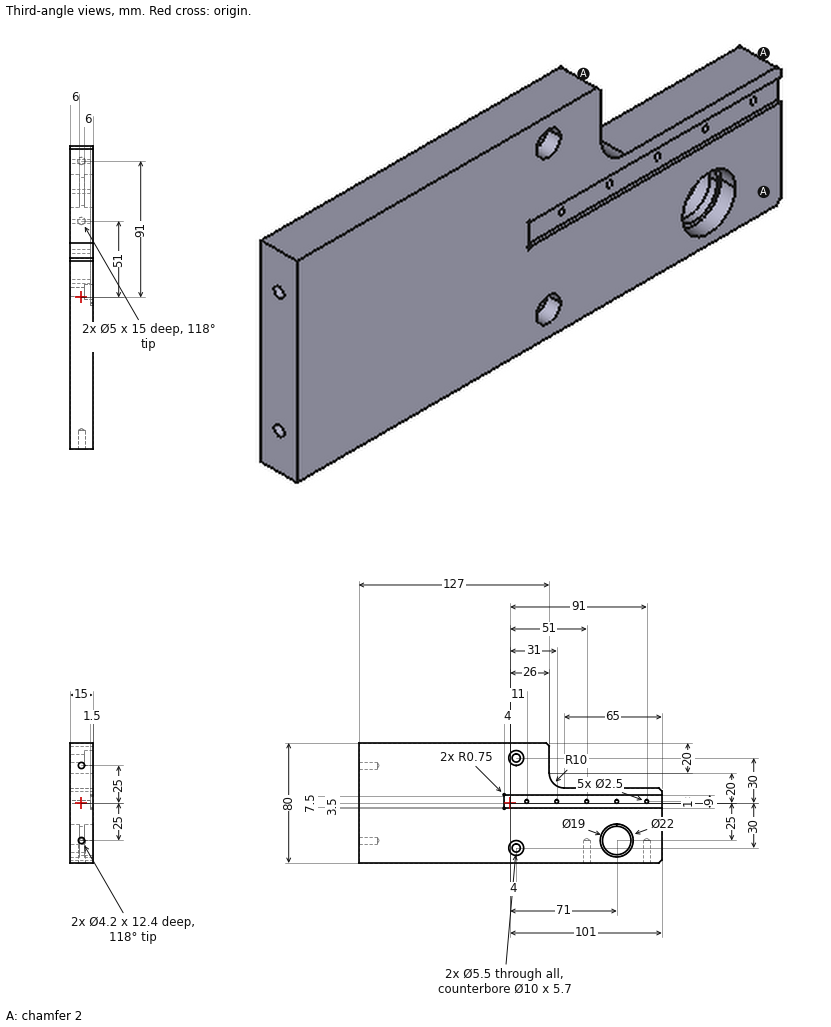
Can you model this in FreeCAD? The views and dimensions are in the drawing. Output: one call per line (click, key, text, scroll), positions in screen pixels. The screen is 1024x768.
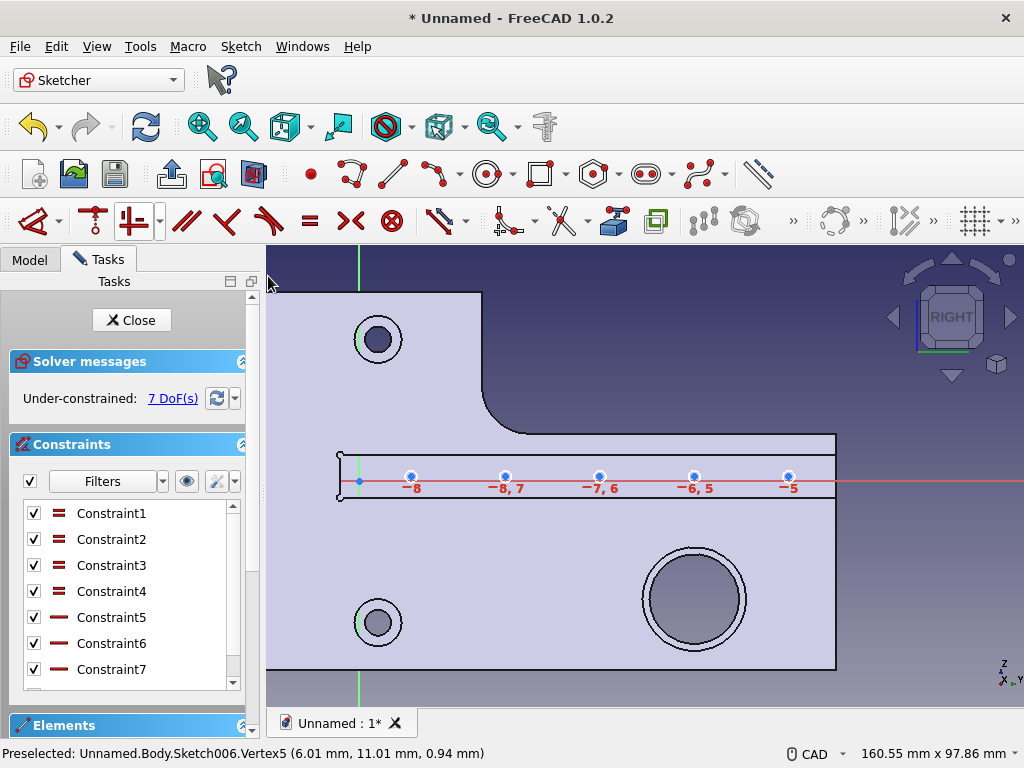
key(d)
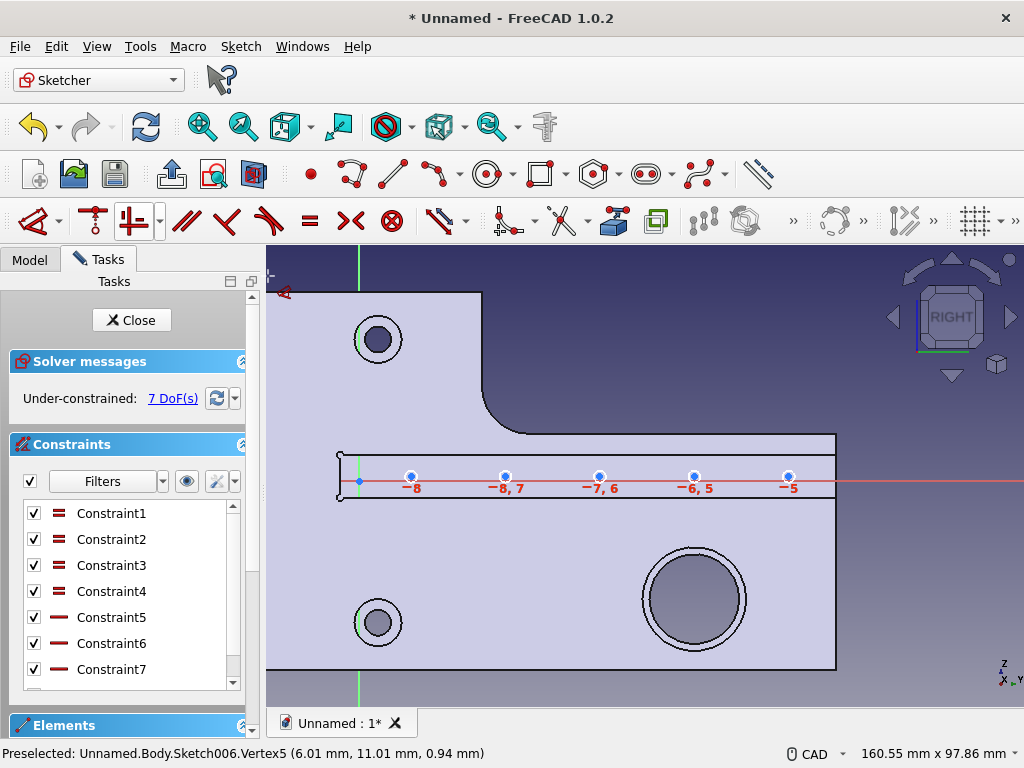
scroll(793, 481, up, 7)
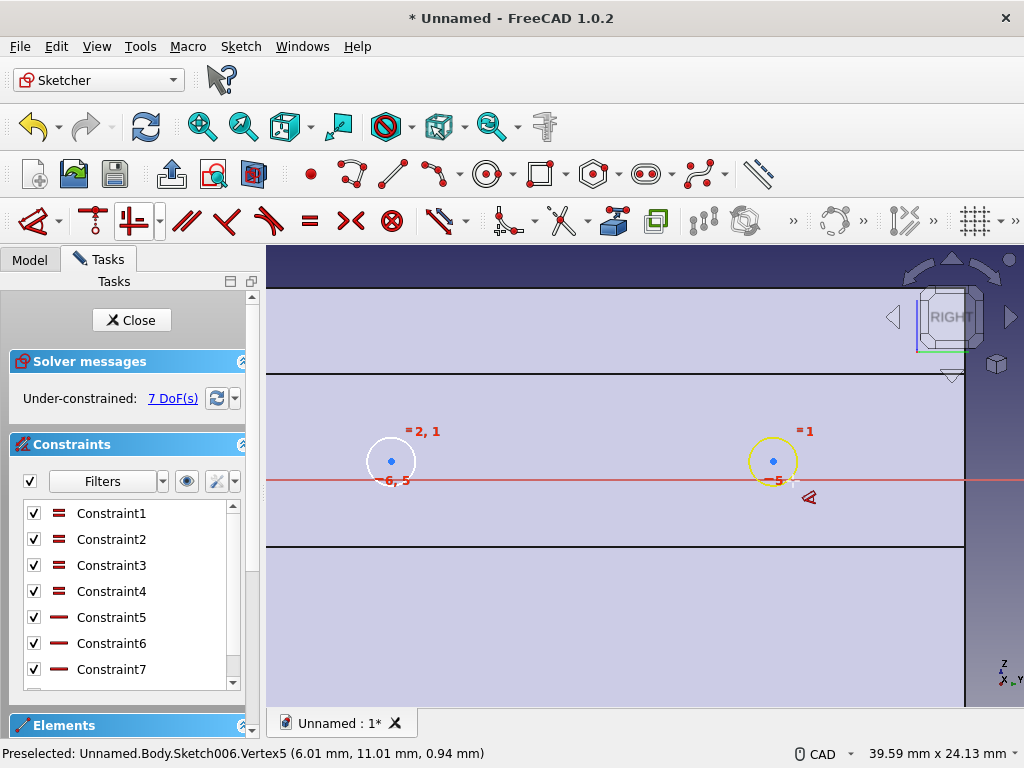
click(790, 479)
click(812, 502)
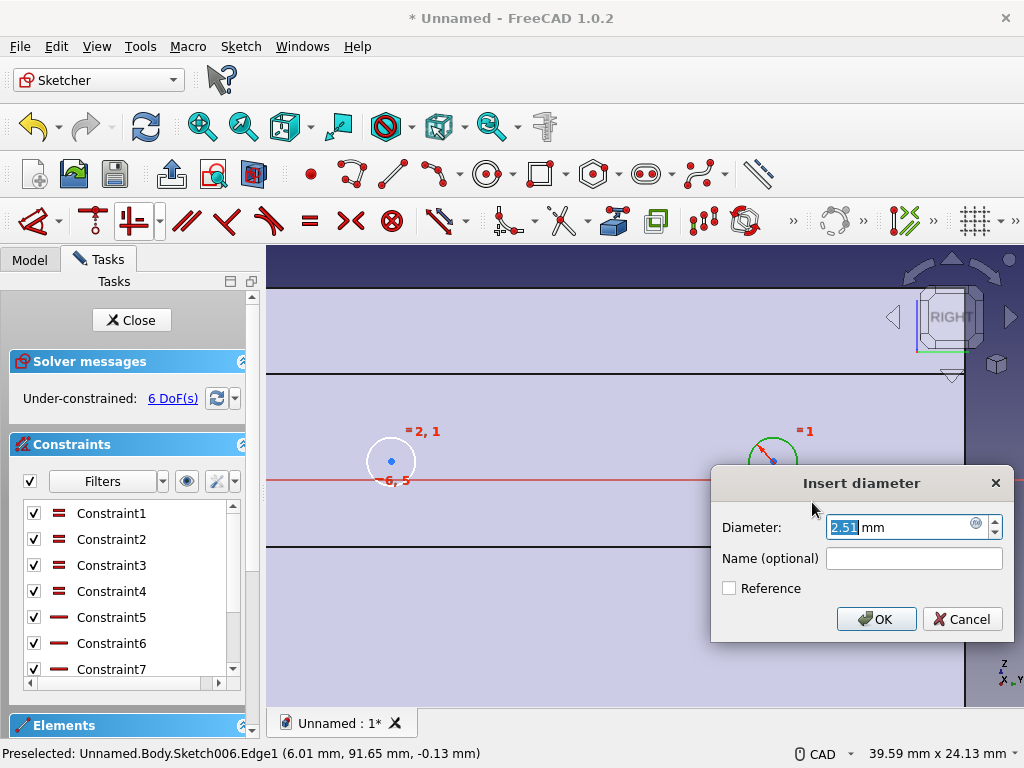
text(2.5)
key(Return)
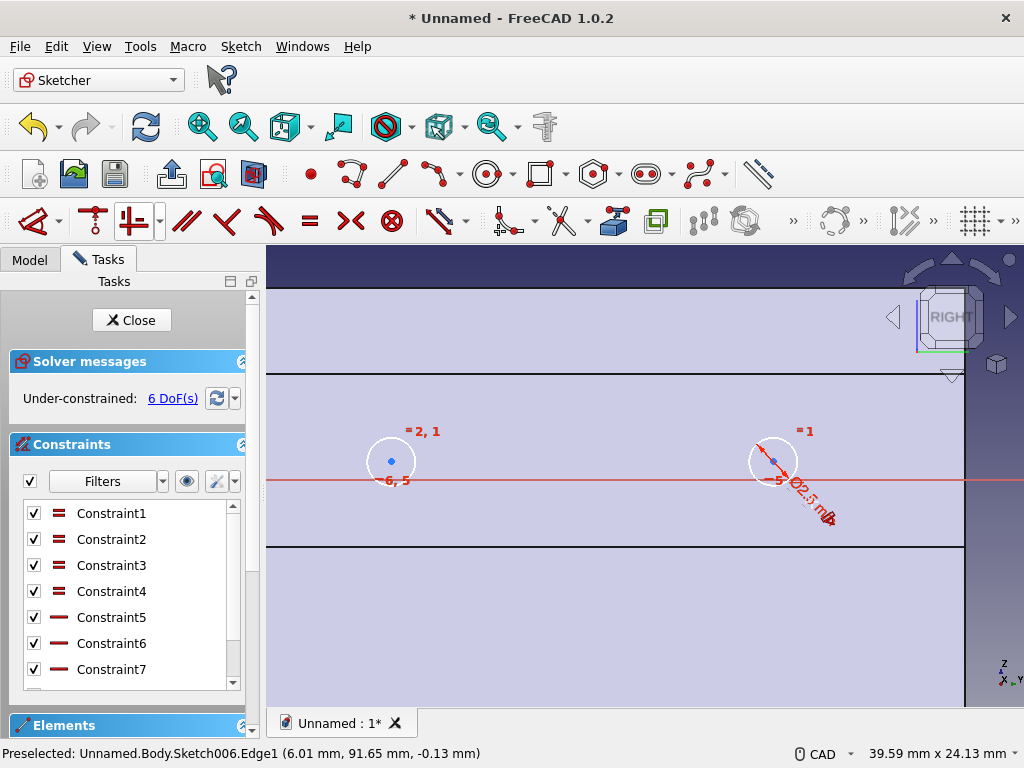
scroll(773, 462, up, 4)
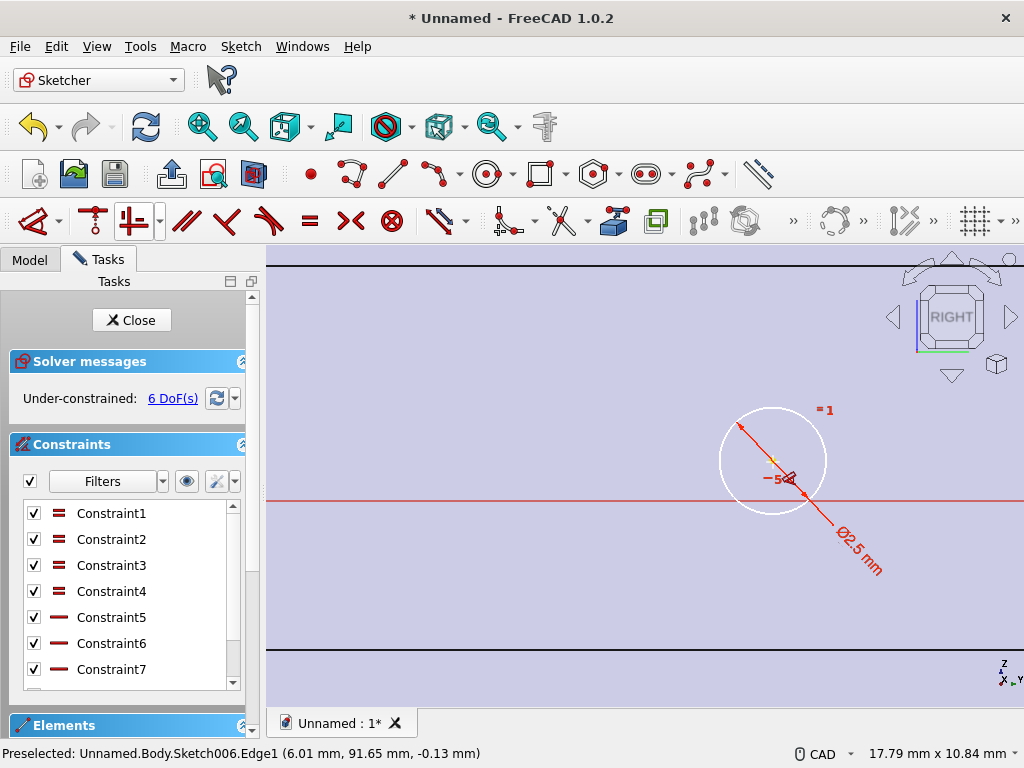
click(773, 461)
click(807, 481)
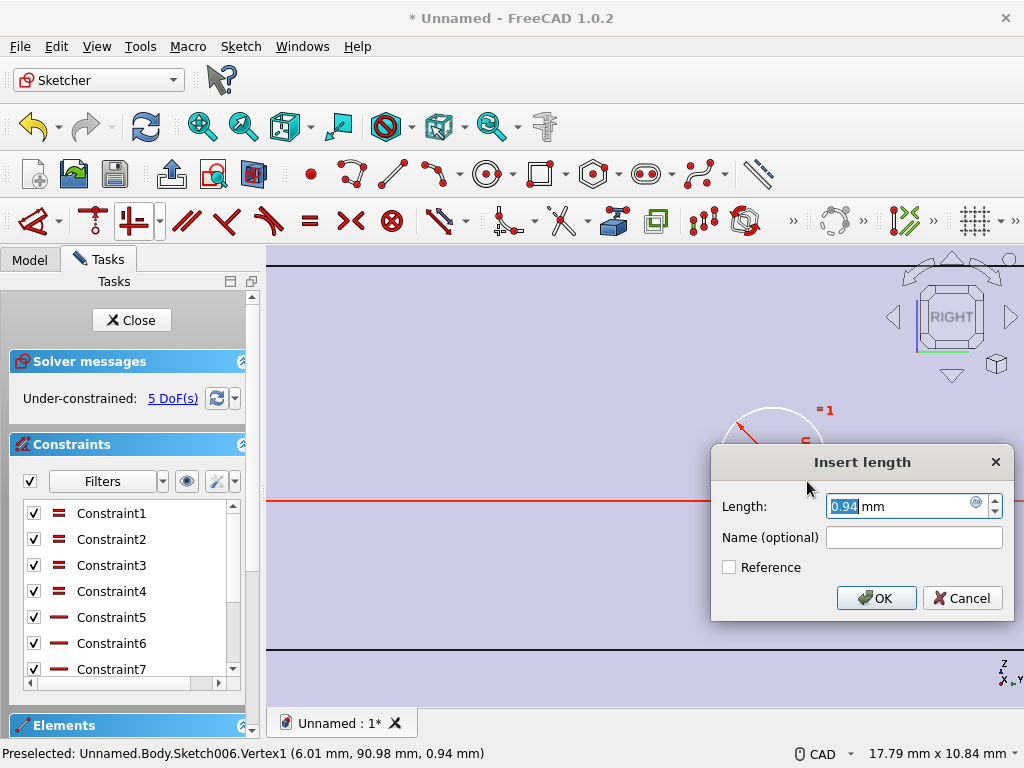
text(1)
key(Return)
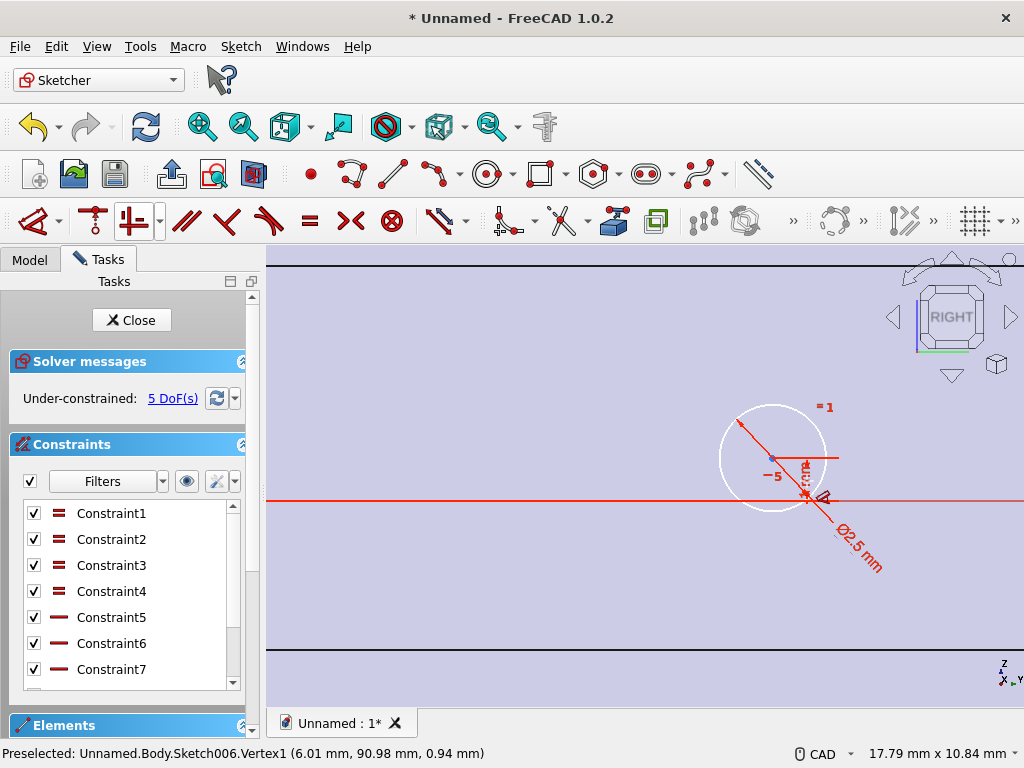
scroll(790, 478, down, 11)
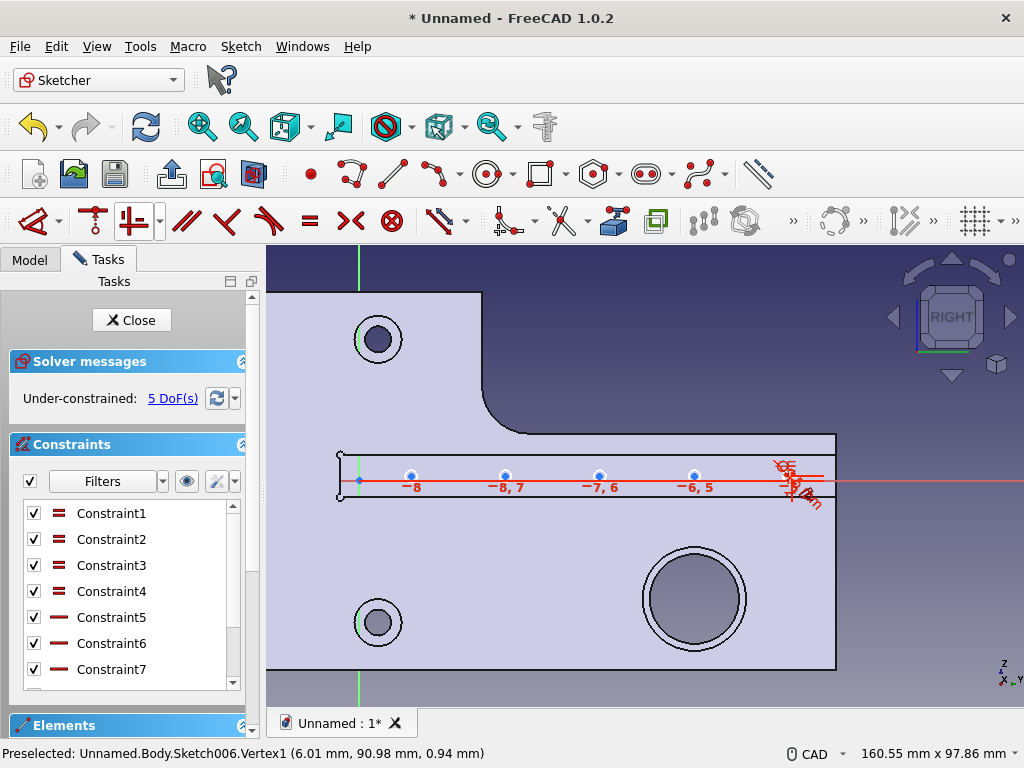
click(789, 476)
click(574, 515)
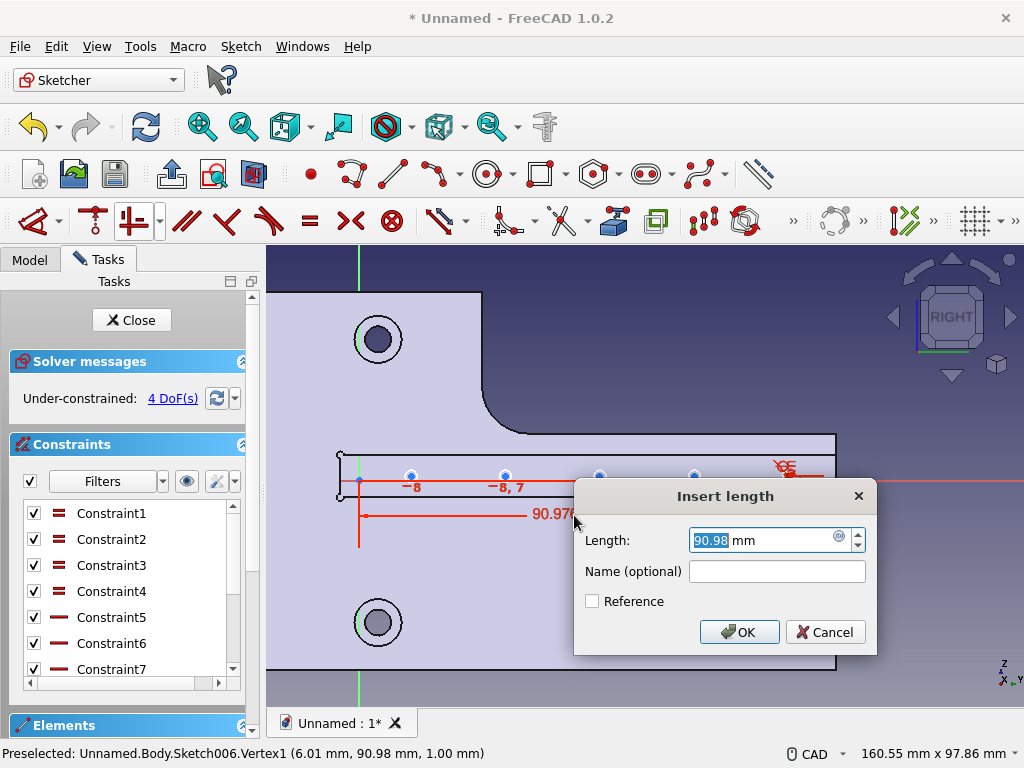
text(91)
key(Return)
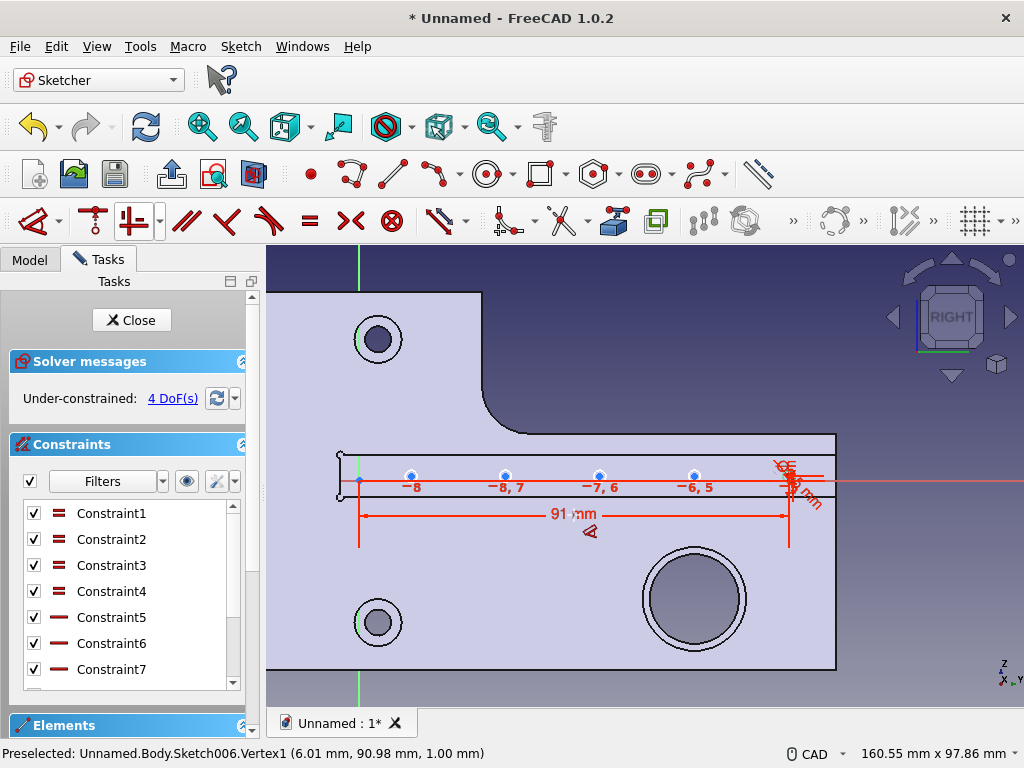
click(695, 476)
click(450, 515)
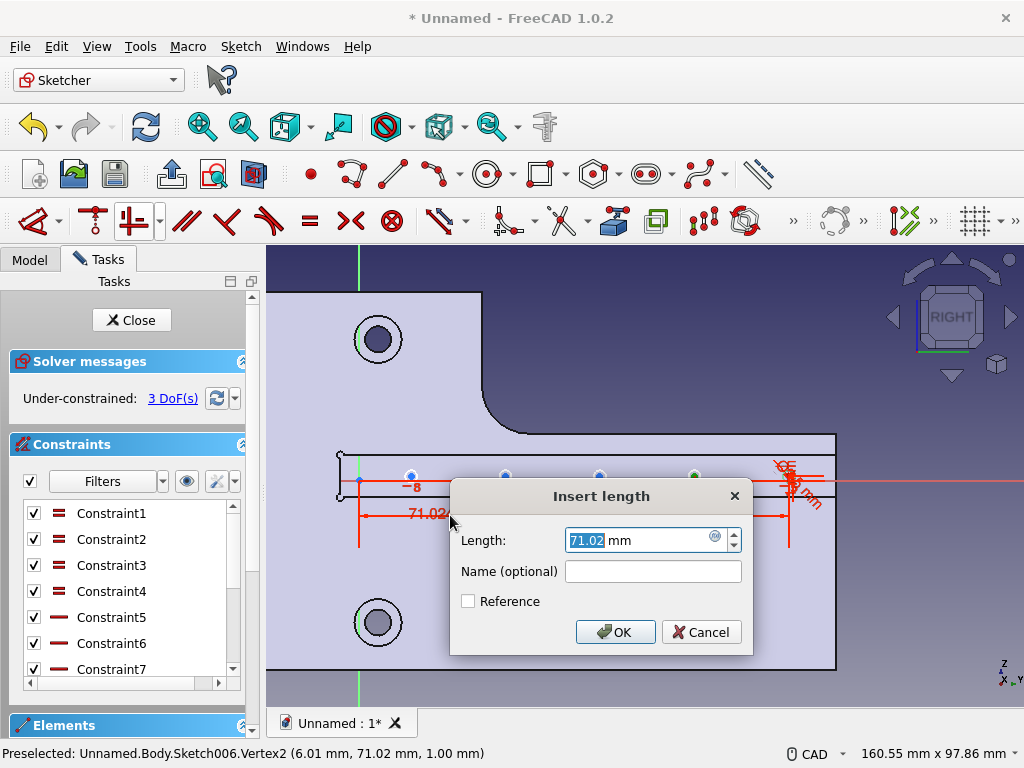
text(71)
key(Return)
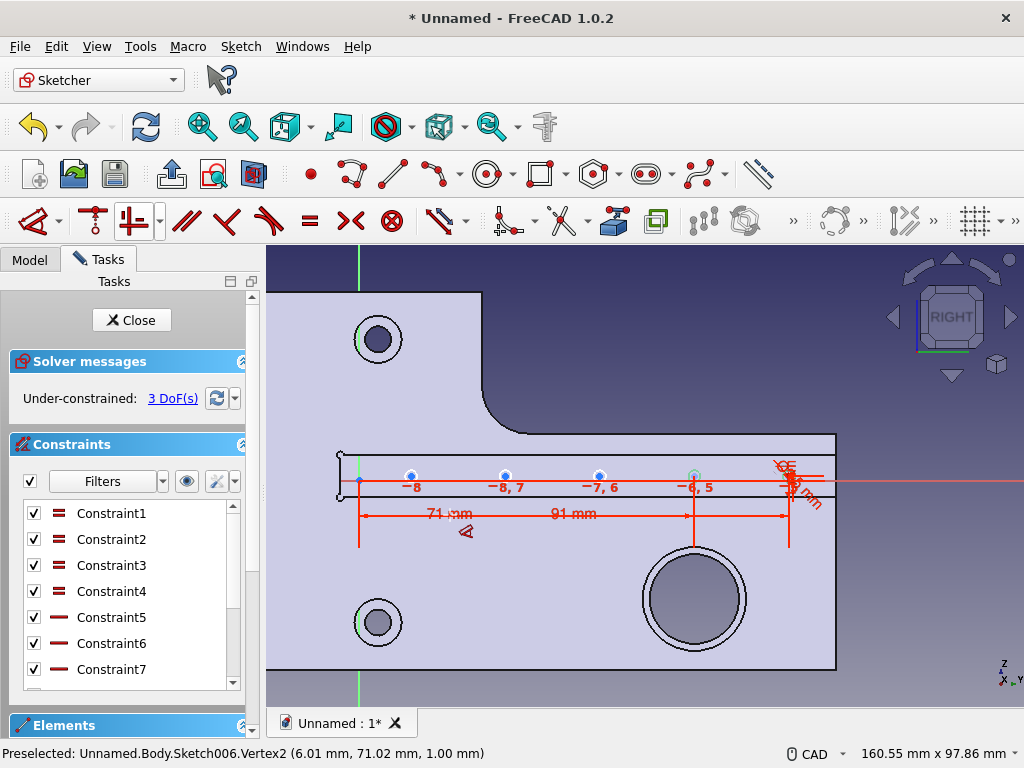
click(600, 476)
click(480, 442)